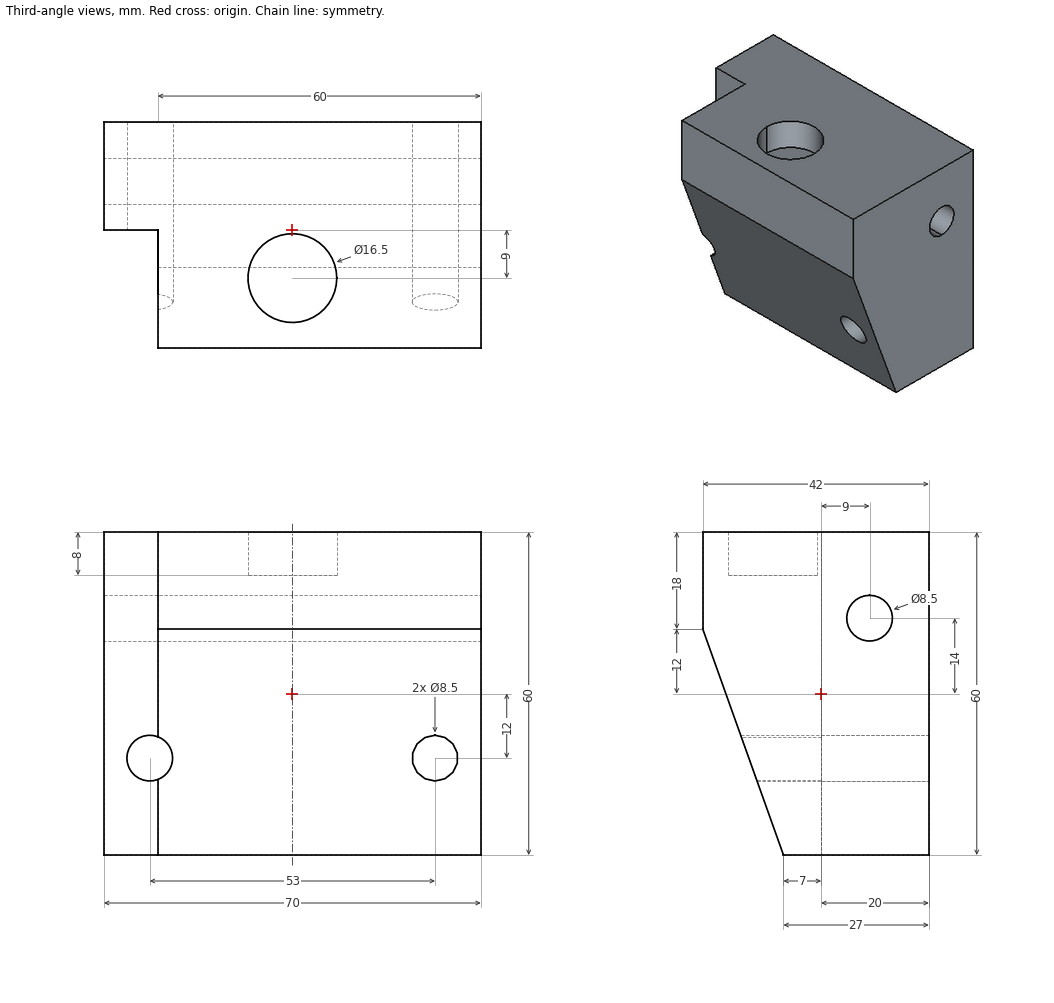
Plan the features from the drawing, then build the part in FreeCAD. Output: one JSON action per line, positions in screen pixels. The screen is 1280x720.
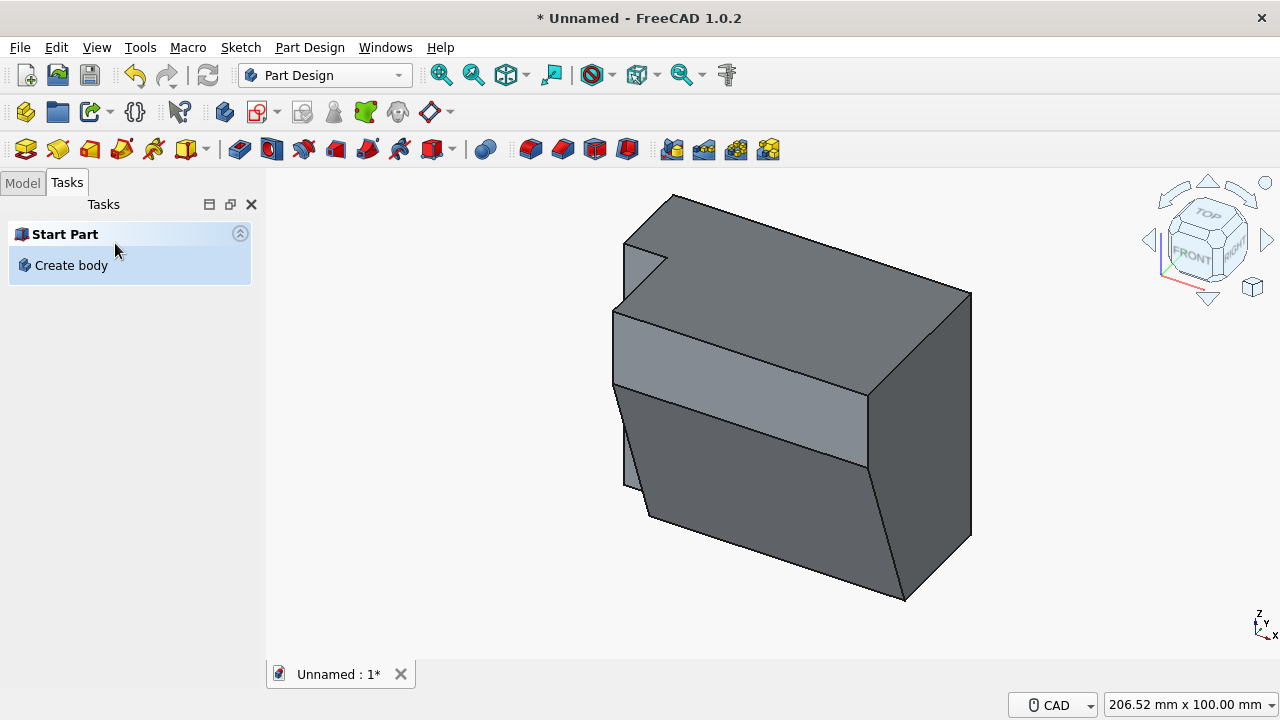
{"action": "key", "text": "6"}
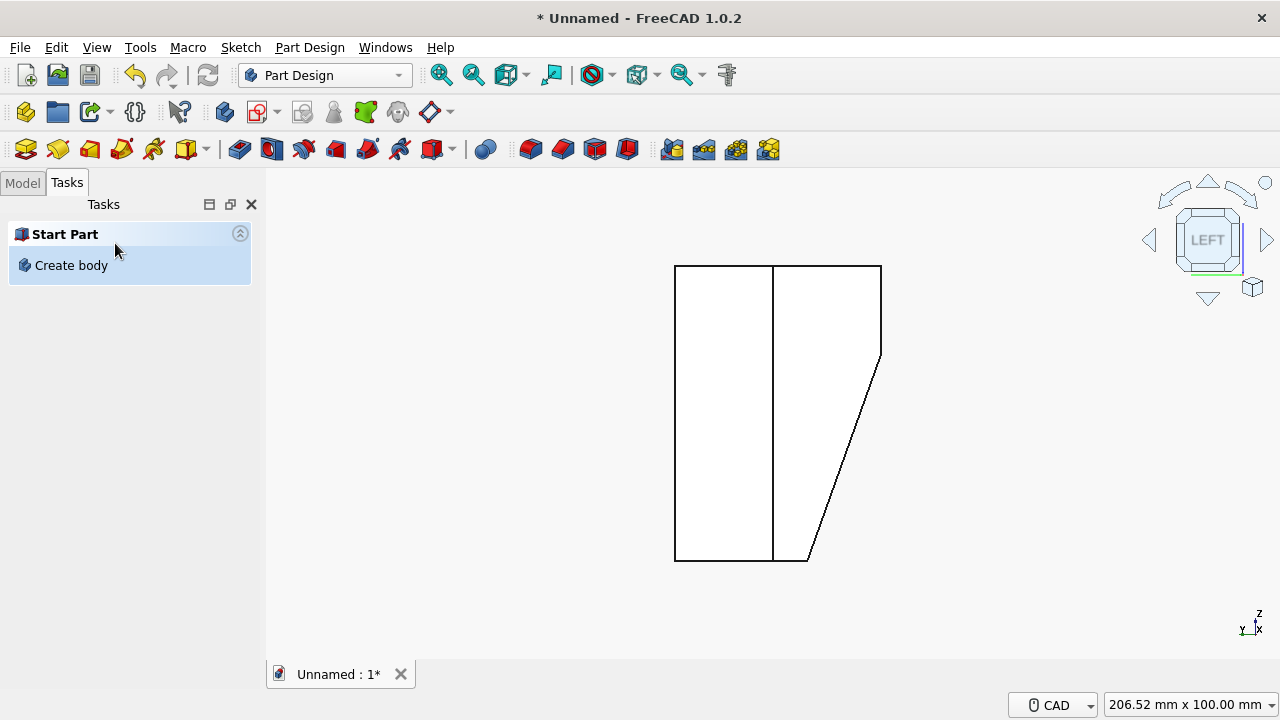
{"action": "left_click", "coordinate": [724, 370]}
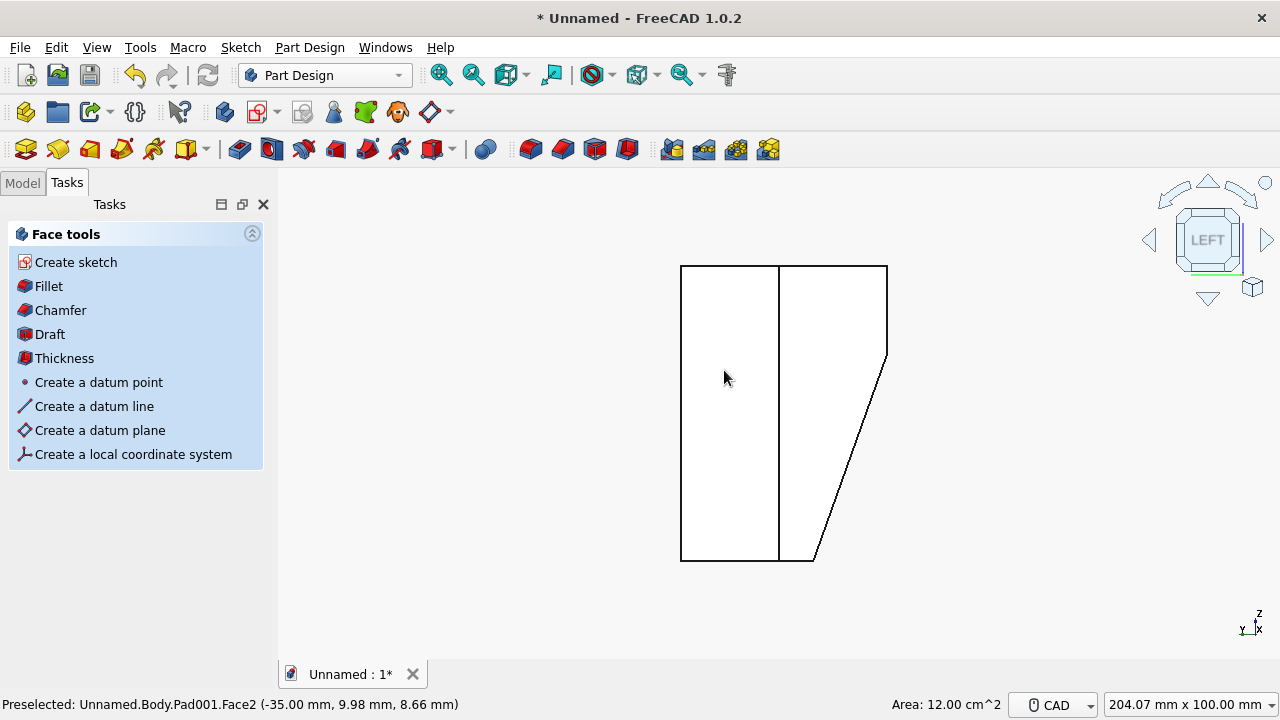
{"action": "left_click", "coordinate": [258, 112]}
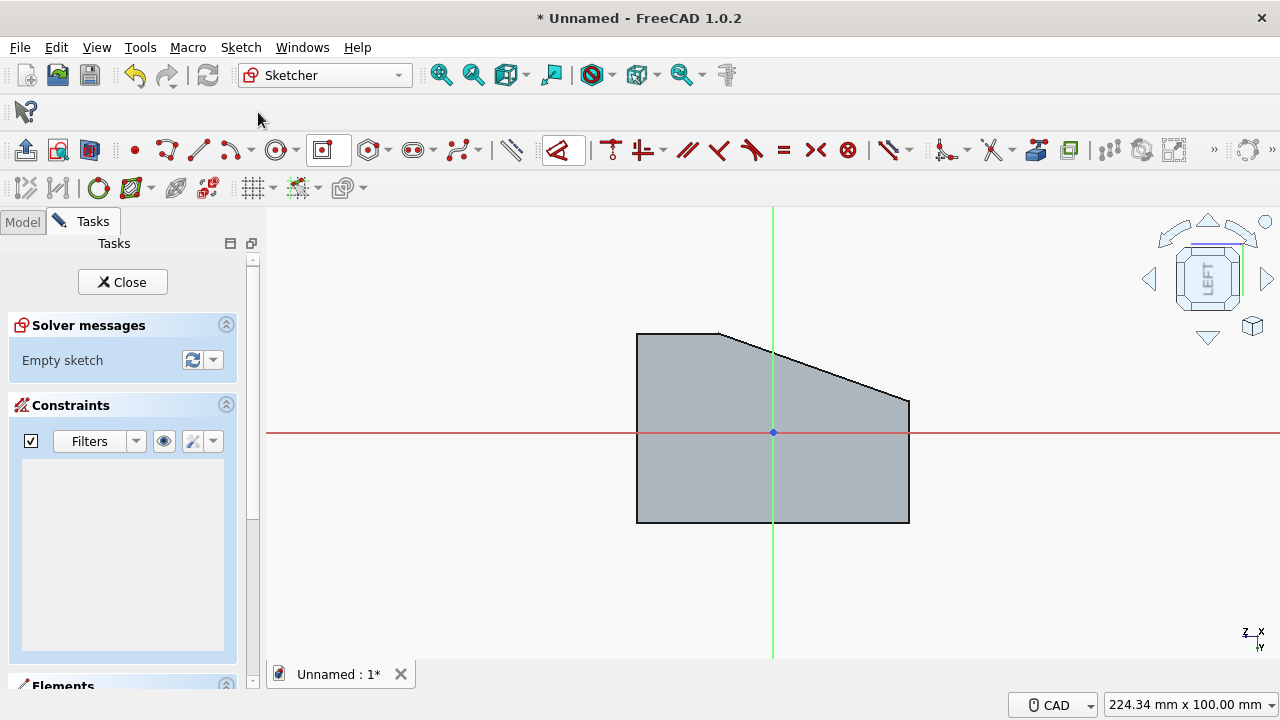
{"action": "scroll", "coordinate": [739, 471], "scroll_direction": "up", "scroll_amount": 8}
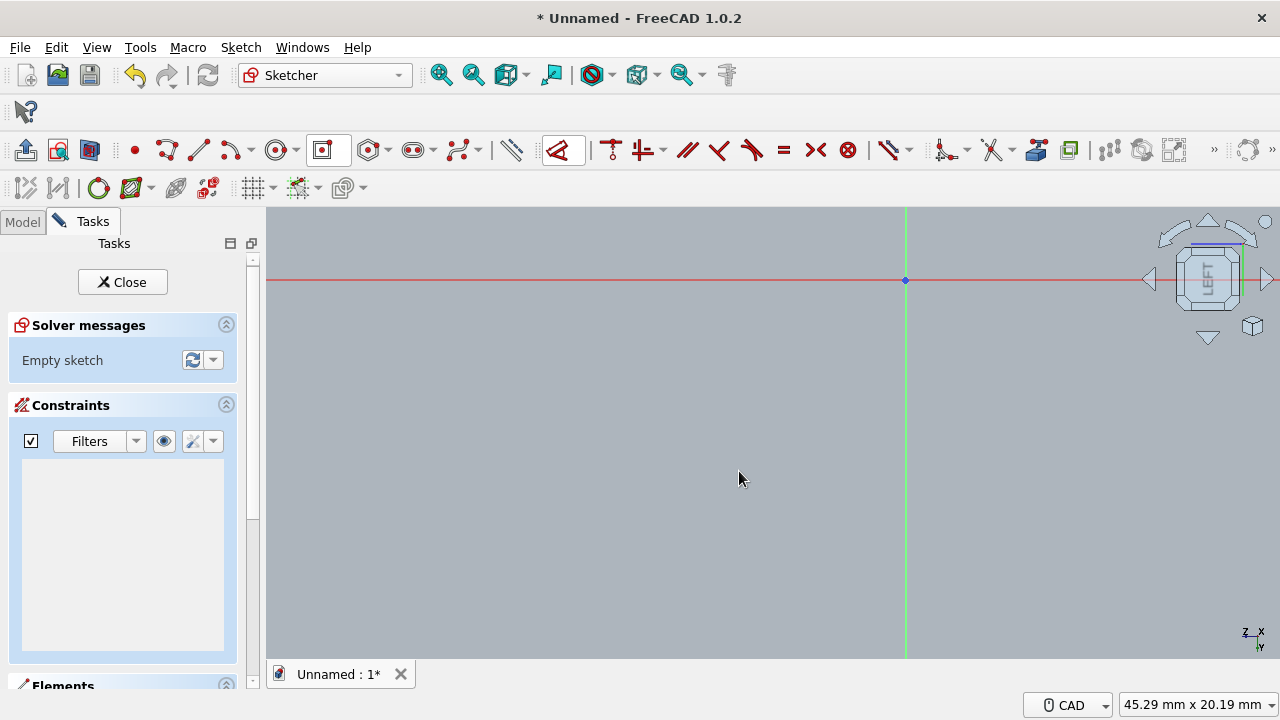
{"action": "key", "text": "g c"}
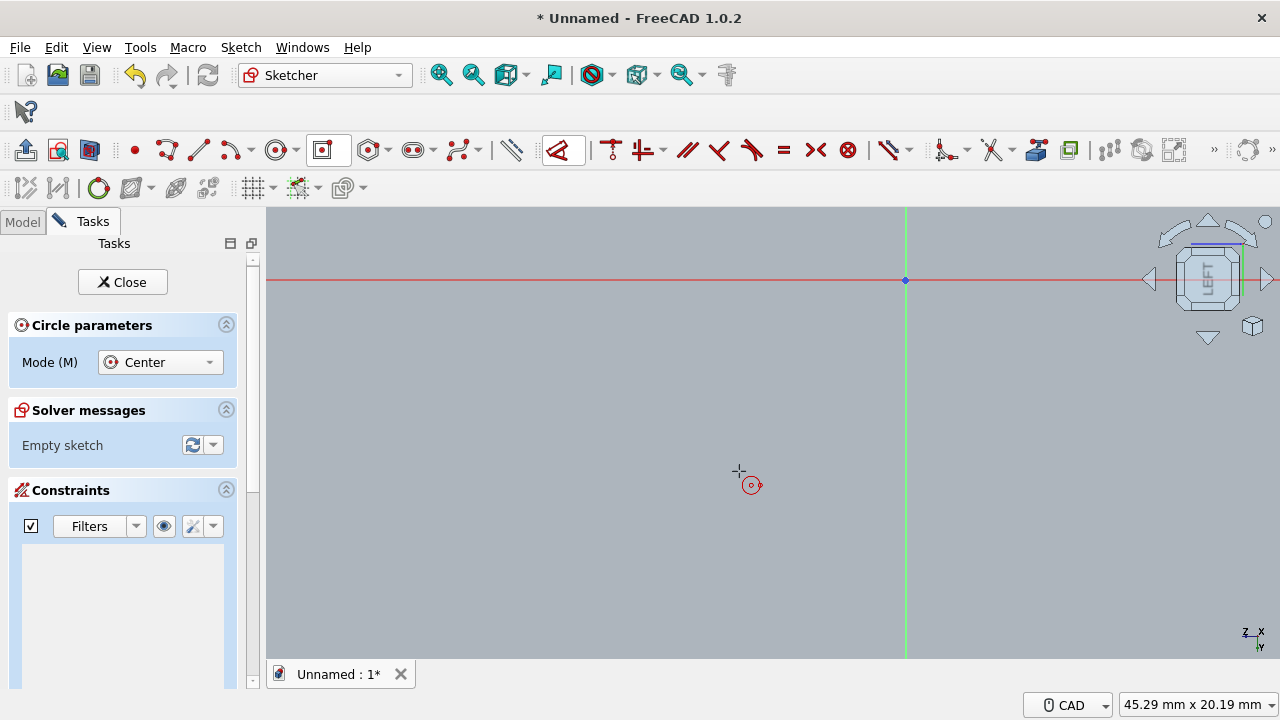
{"action": "left_click", "coordinate": [592, 482]}
{"action": "mouse_move", "coordinate": [659, 415]}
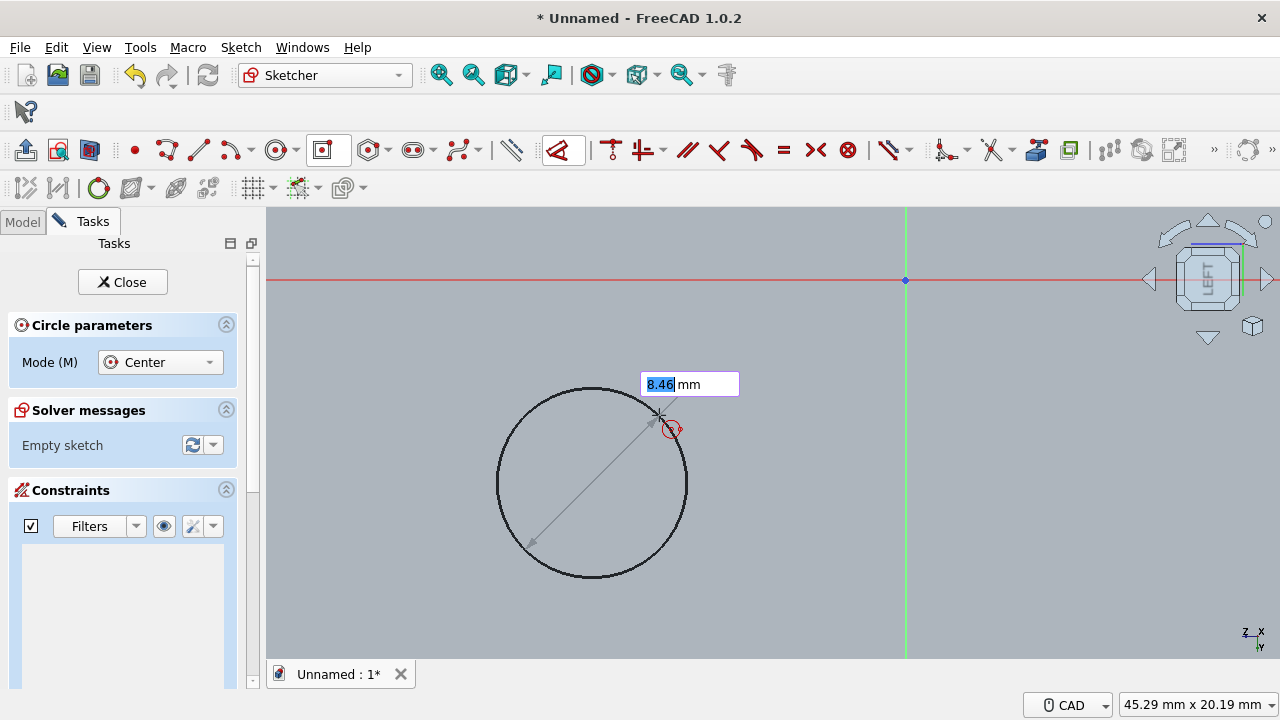
{"action": "type", "text": "8.5"}
{"action": "key", "text": "Return"}
{"action": "key", "text": "Escape"}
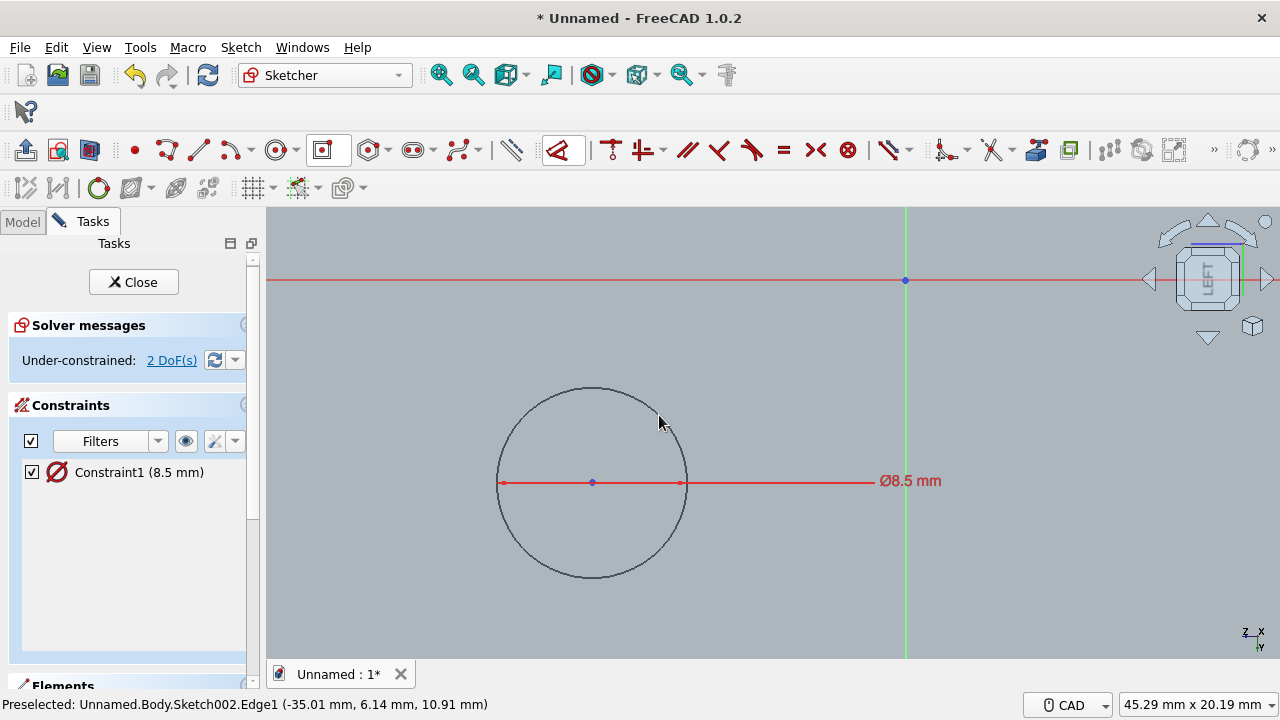
{"action": "left_click", "coordinate": [592, 483]}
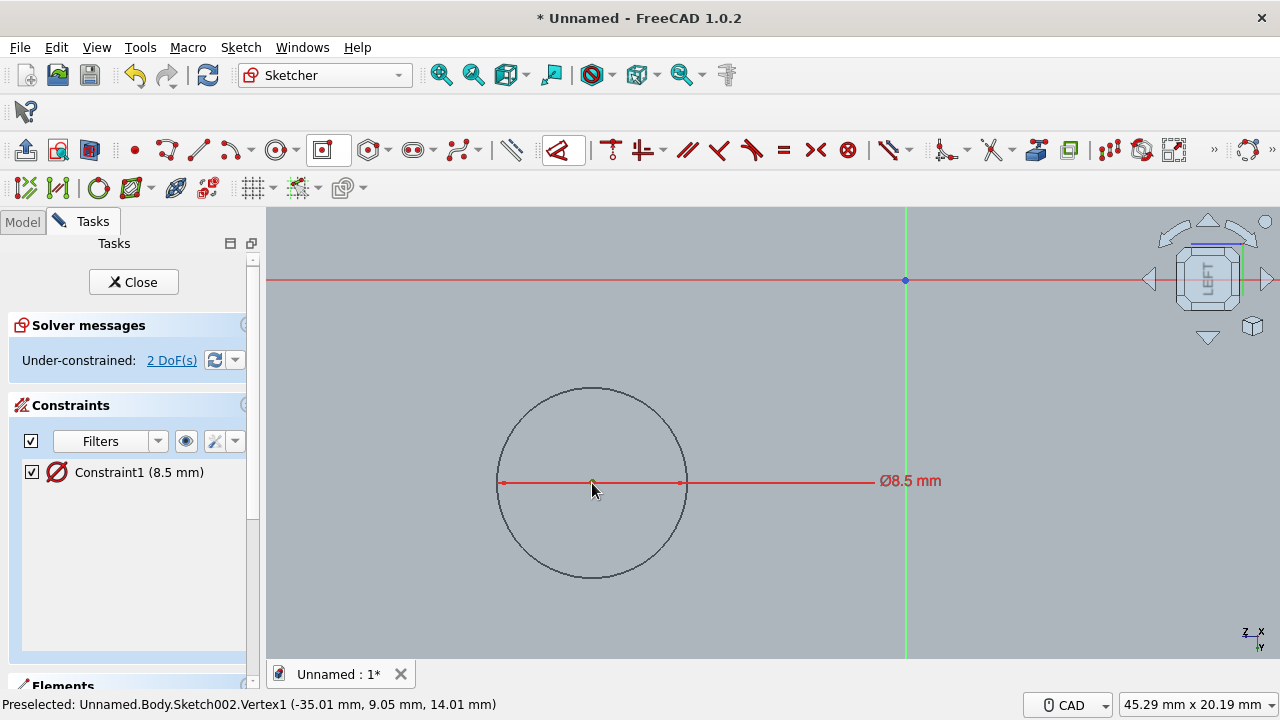
{"action": "key", "text": "i"}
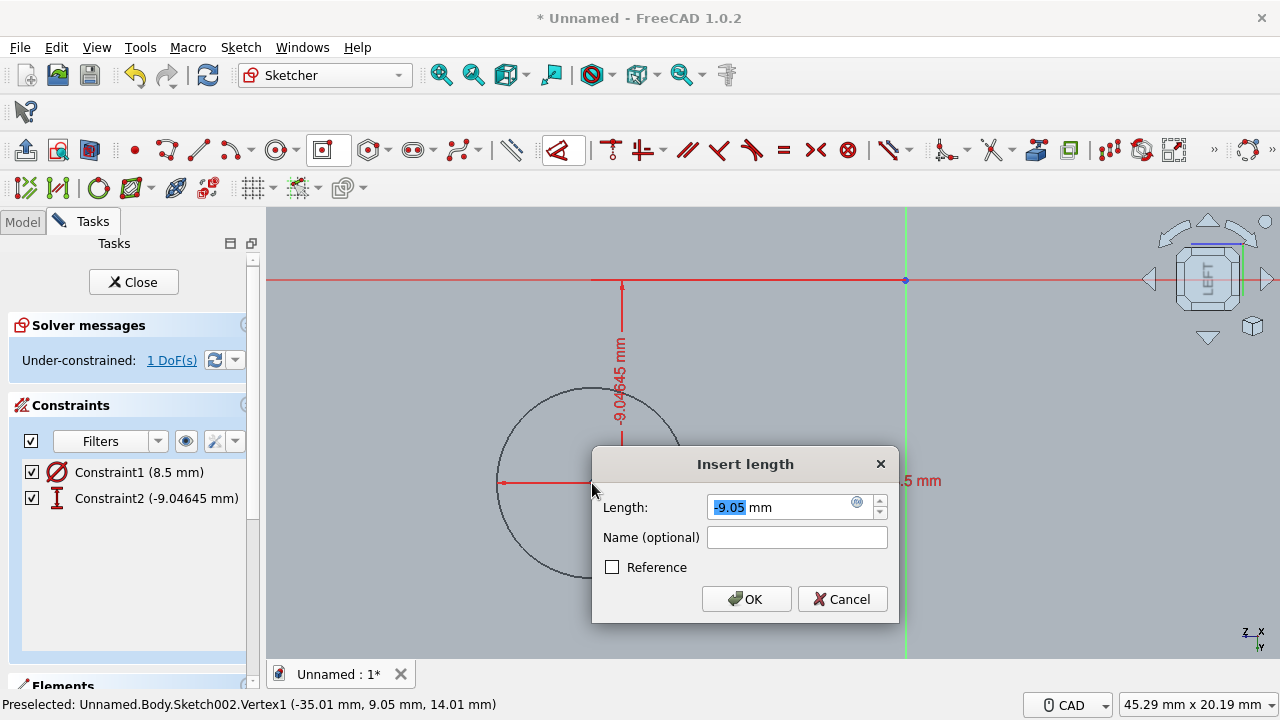
{"action": "type", "text": "-9"}
{"action": "key", "text": "Return"}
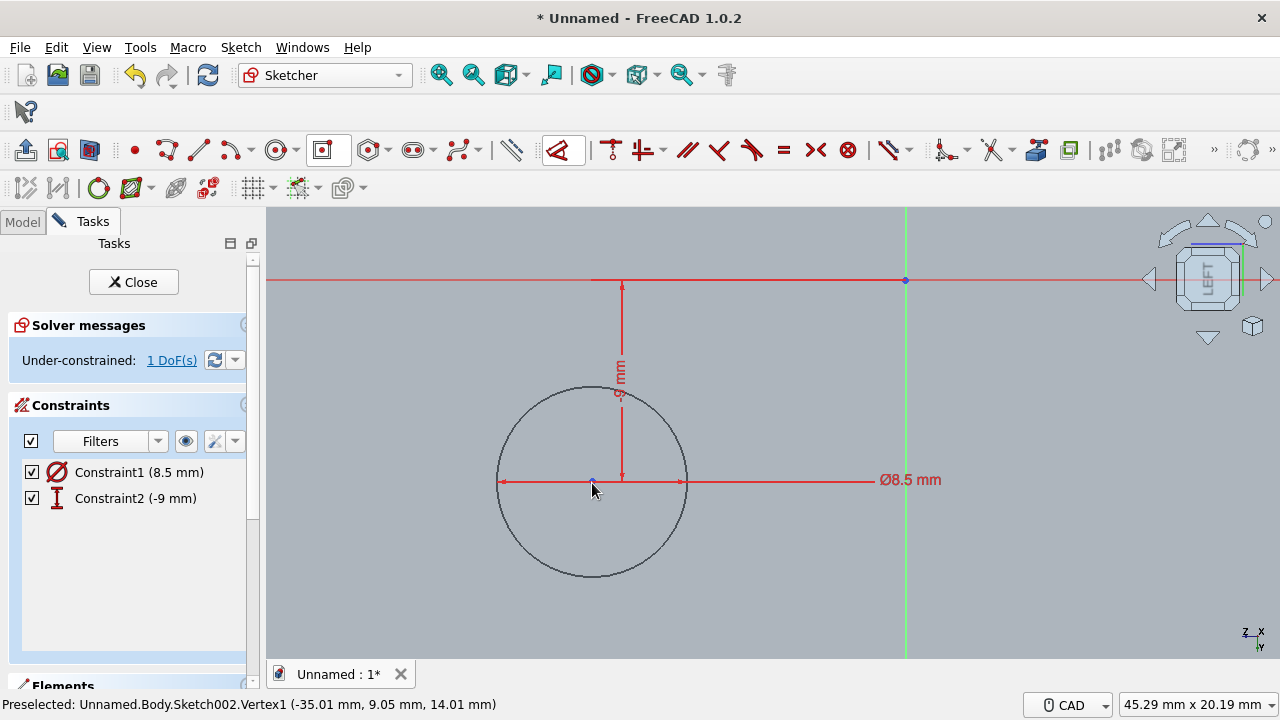
{"action": "left_click", "coordinate": [592, 482]}